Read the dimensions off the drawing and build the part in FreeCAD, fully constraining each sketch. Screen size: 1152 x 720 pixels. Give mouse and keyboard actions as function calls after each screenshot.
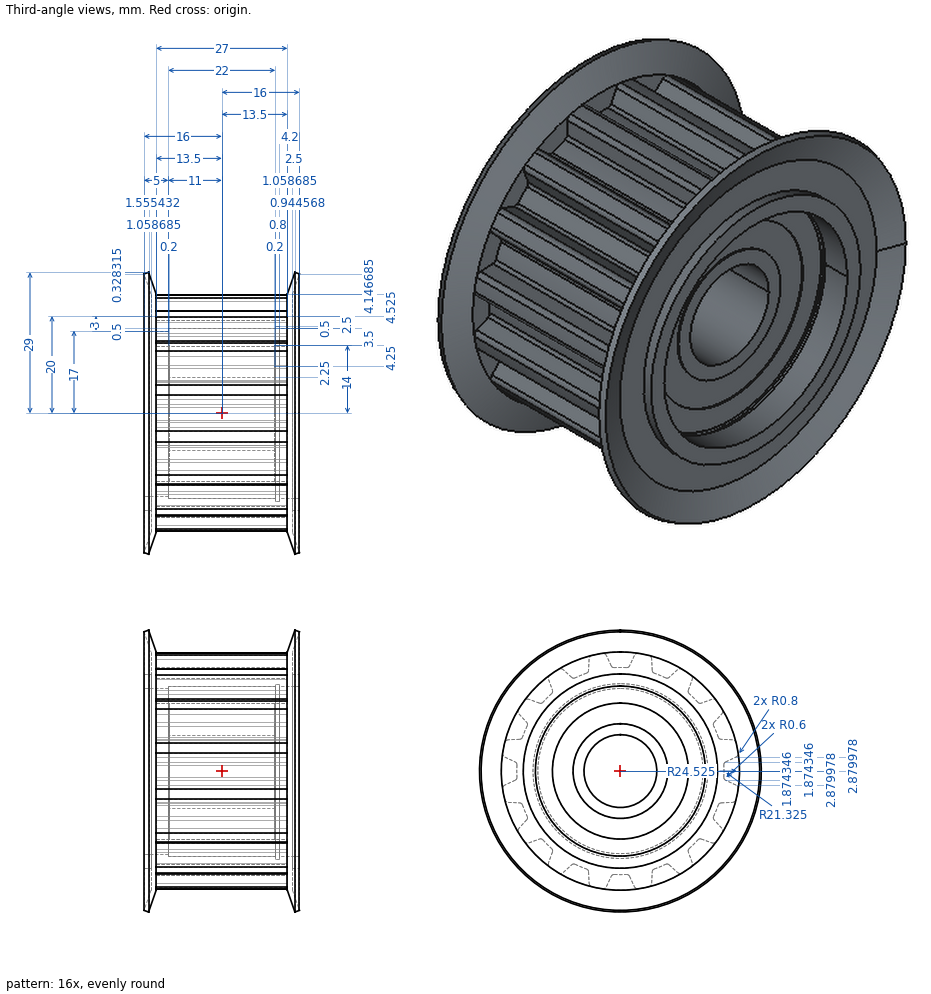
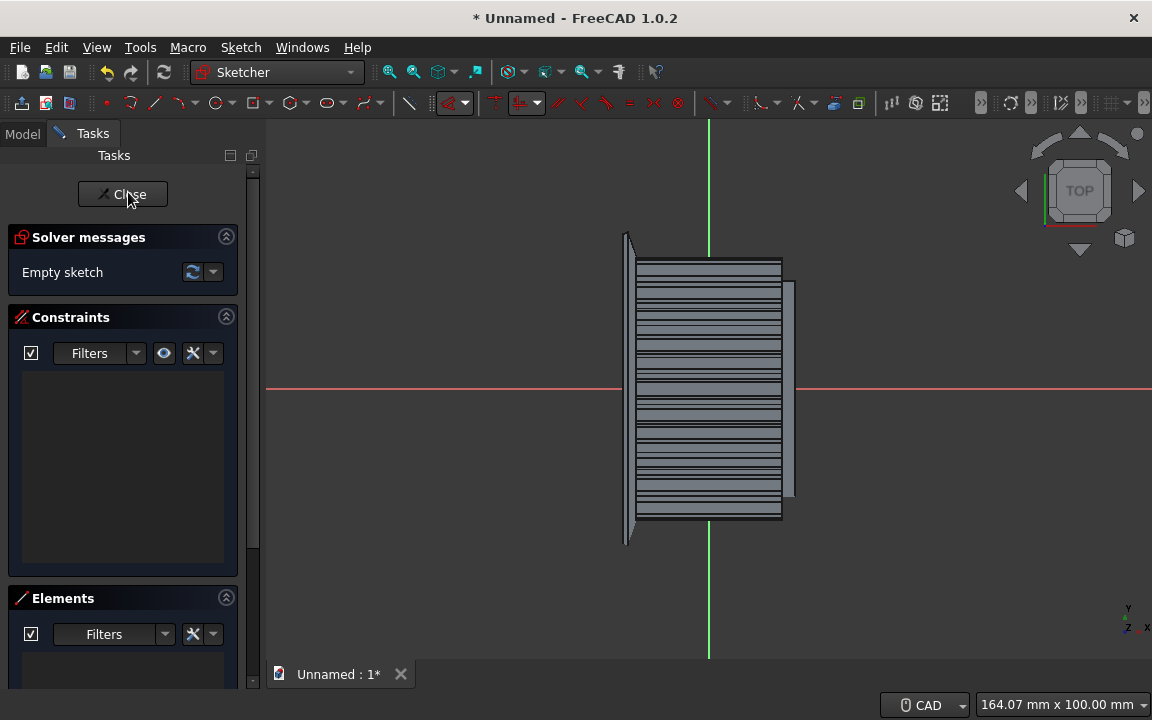
click(70, 104)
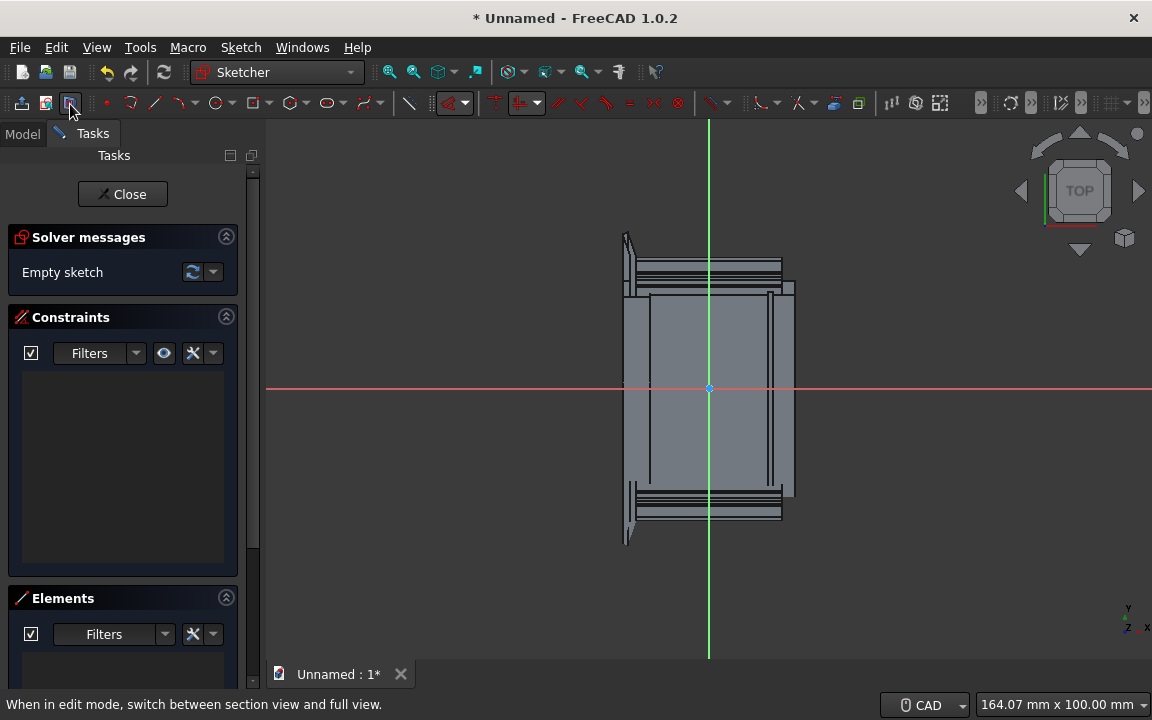
scroll(812, 236, up, 10)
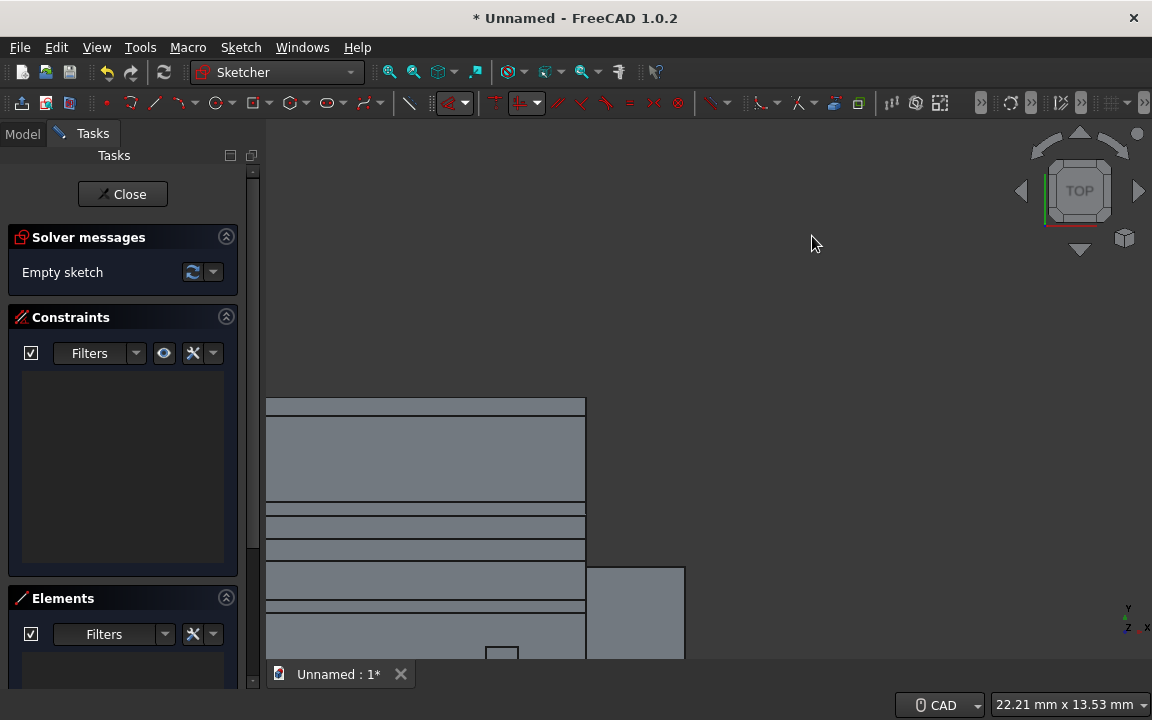
click(132, 104)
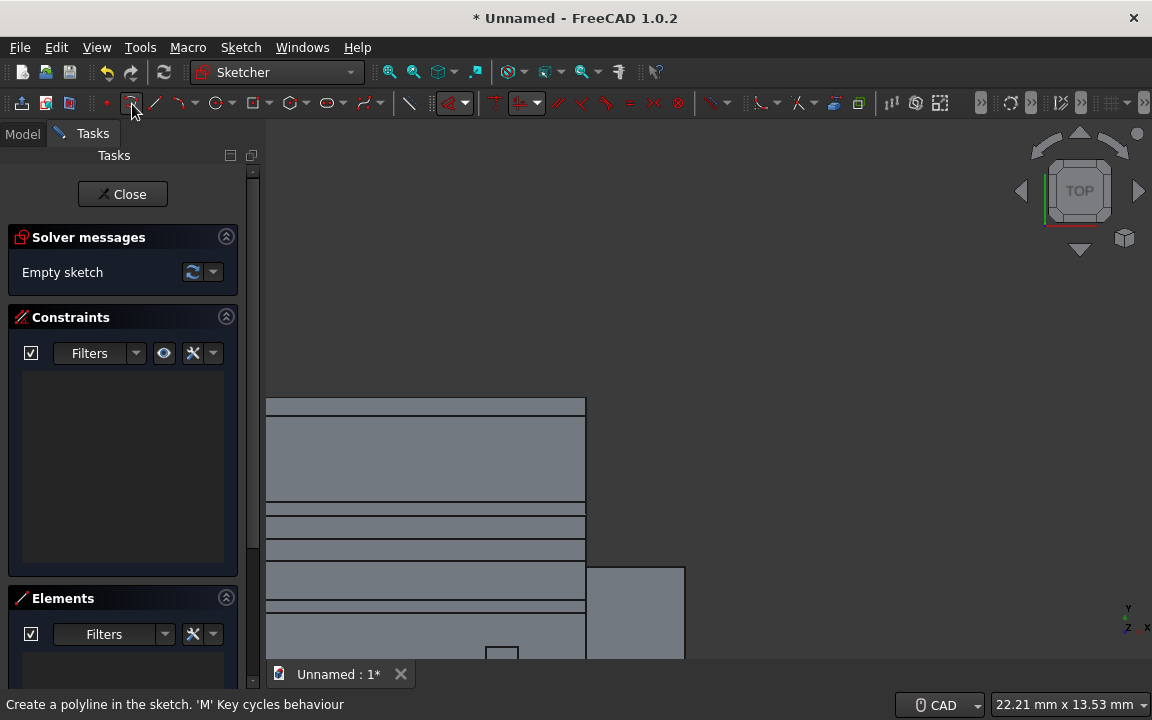
click(586, 567)
click(628, 567)
click(628, 387)
click(685, 221)
click(648, 208)
click(586, 387)
click(586, 568)
key(Escape)
key(Escape)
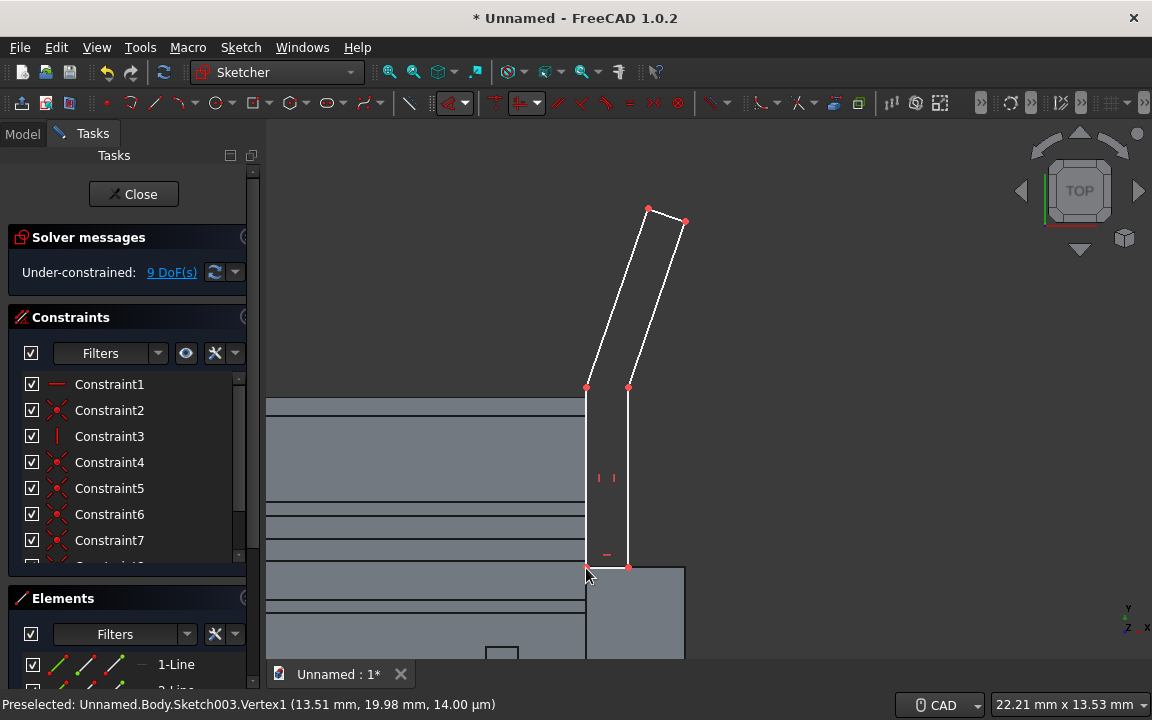
click(586, 568)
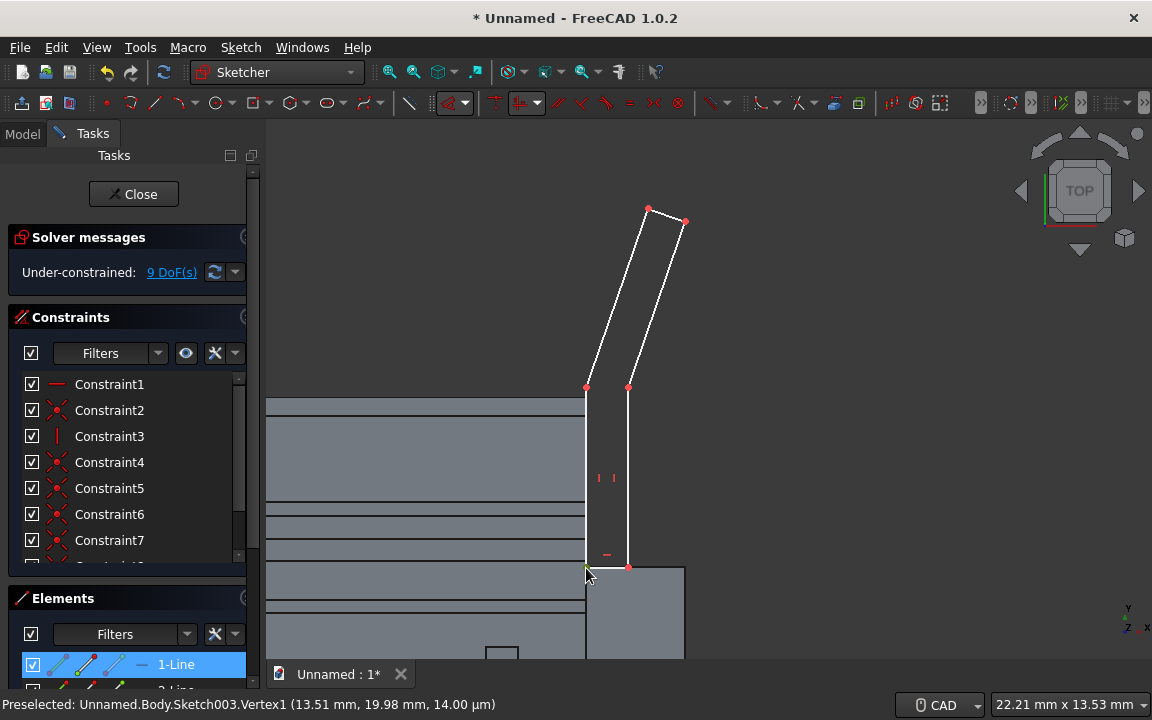
click(468, 104)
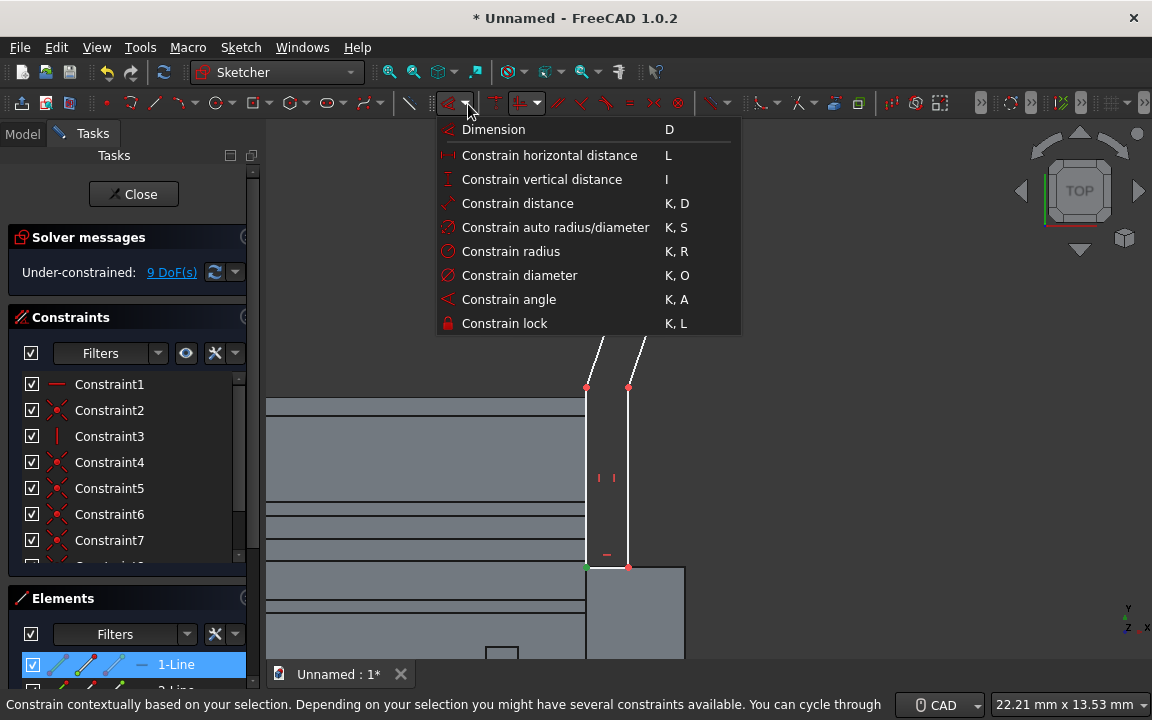
click(589, 179)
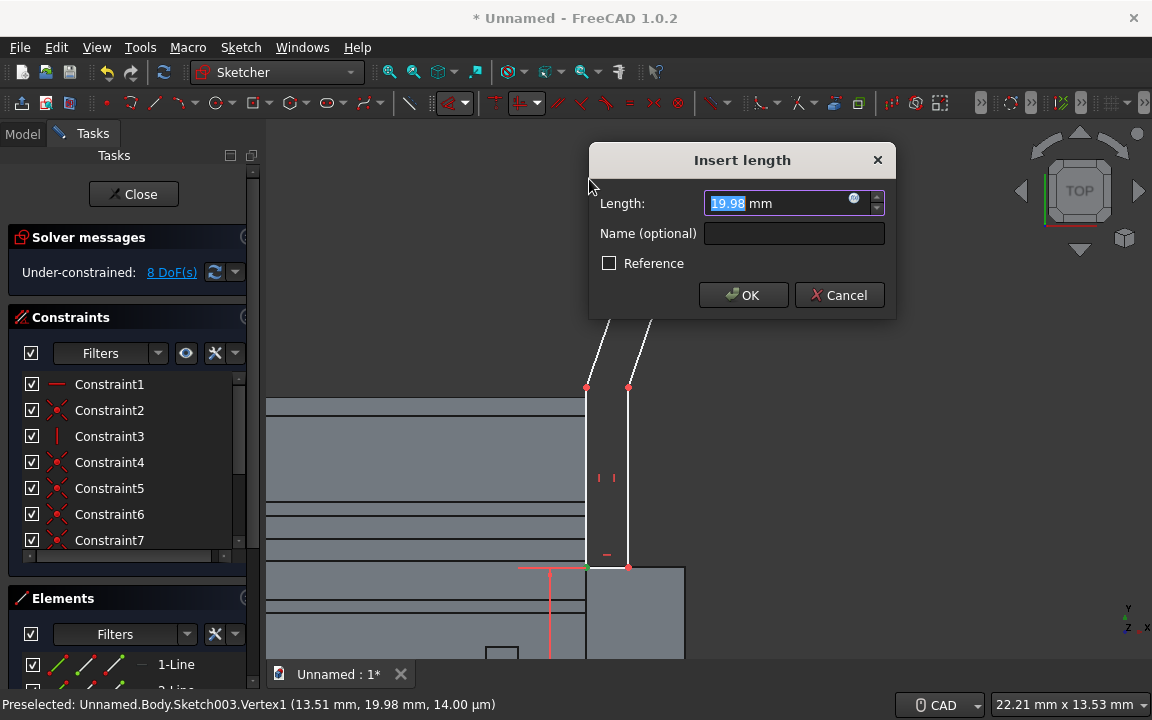
text(20)
key(Return)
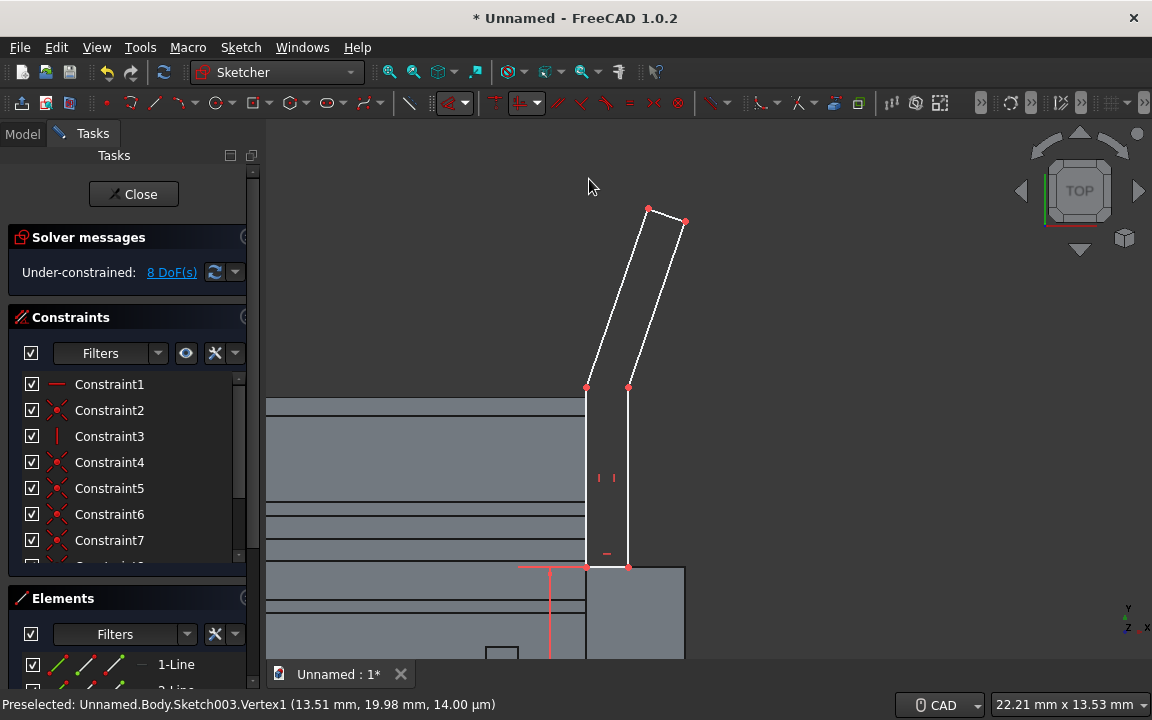
click(685, 222)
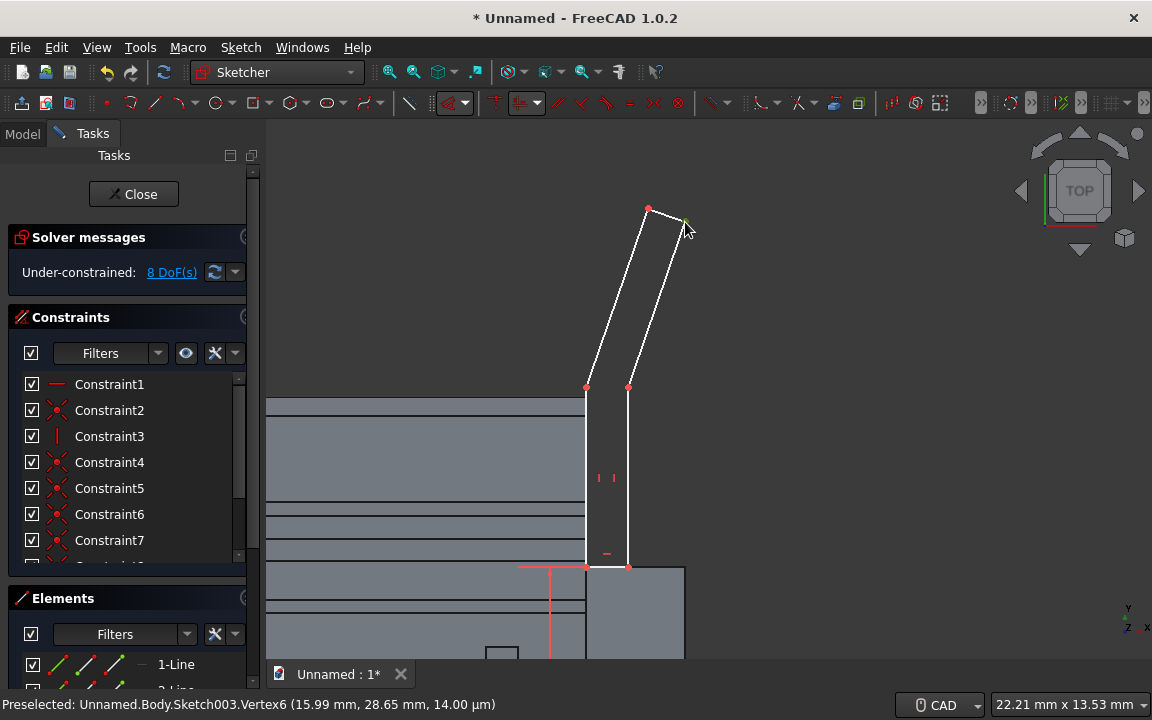
click(468, 104)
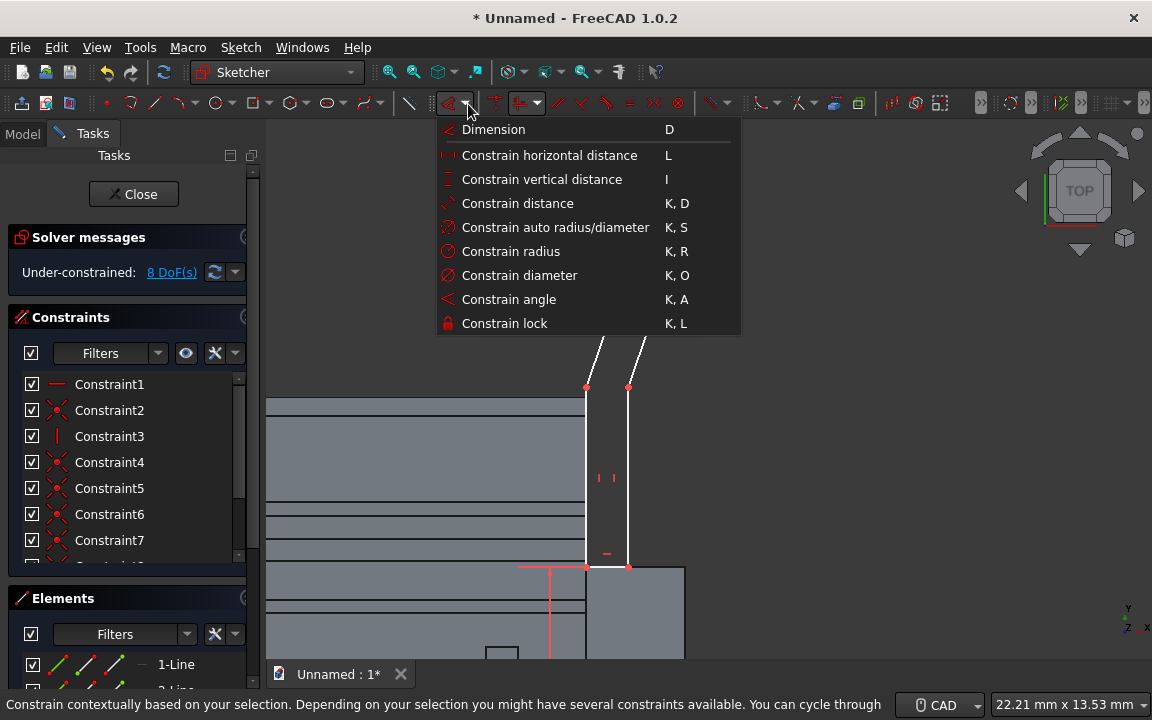
click(589, 155)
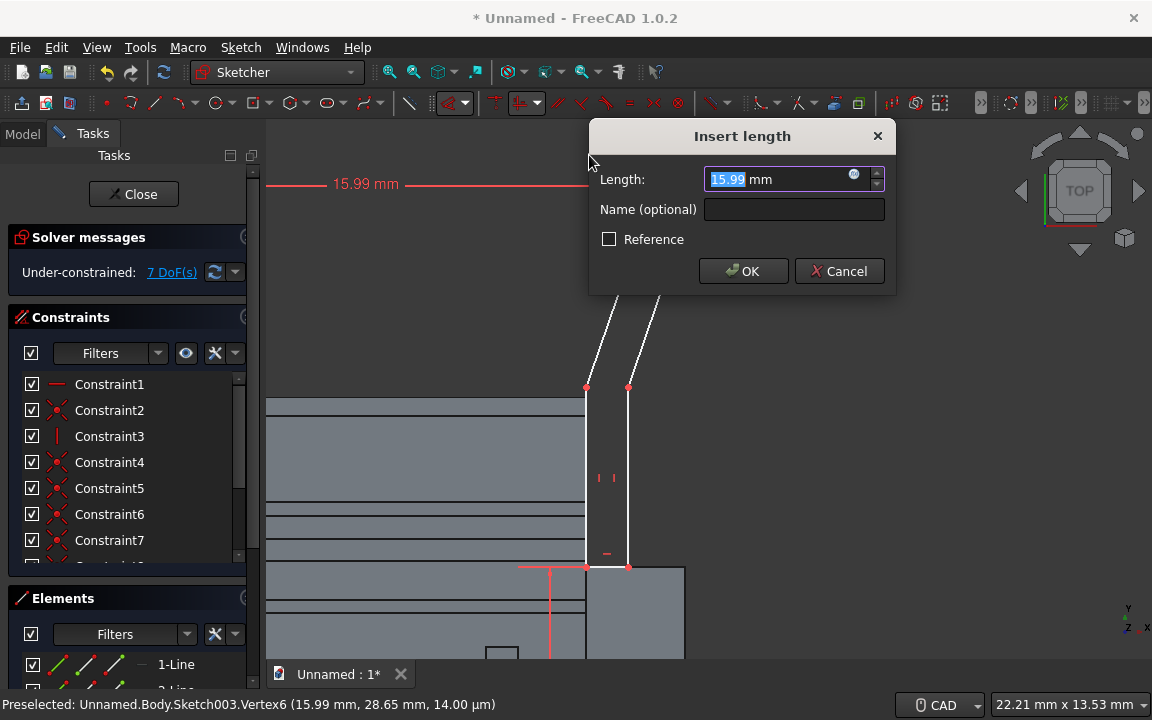
text(16)
key(Return)